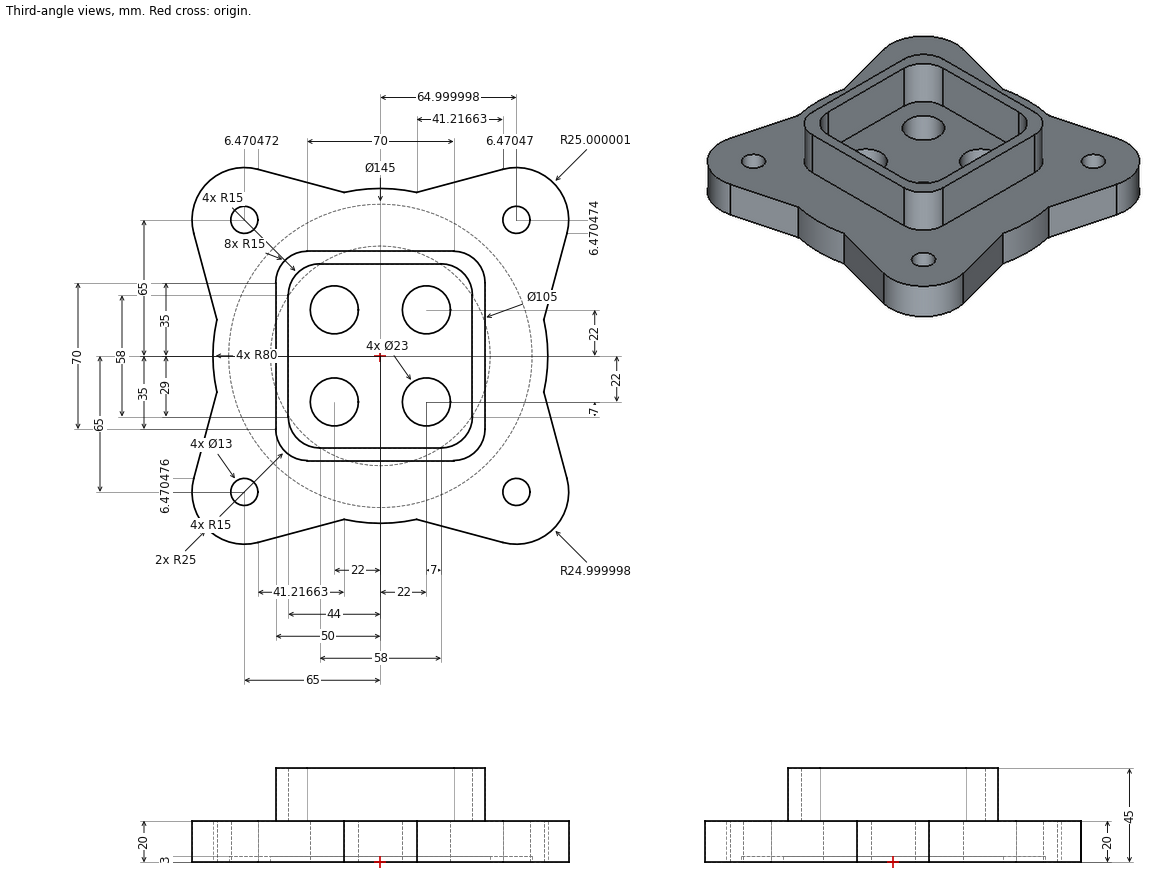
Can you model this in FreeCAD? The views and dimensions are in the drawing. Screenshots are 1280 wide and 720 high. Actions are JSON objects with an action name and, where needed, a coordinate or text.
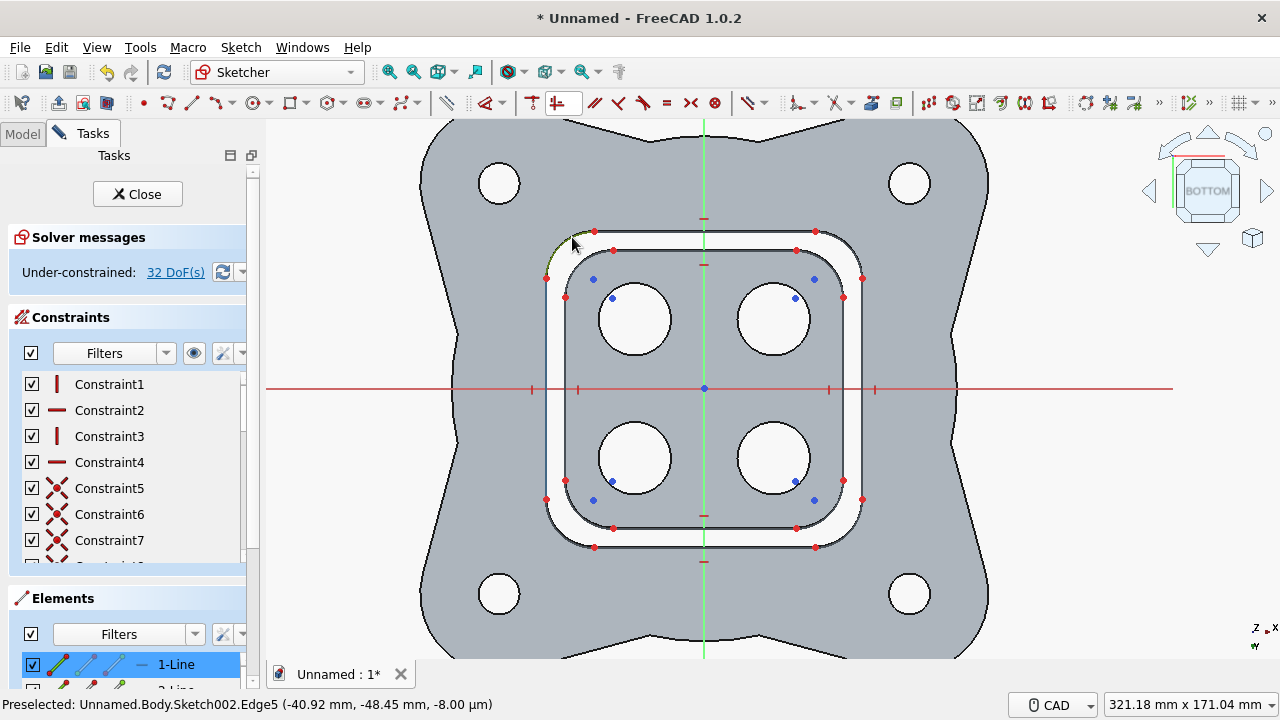
{"action": "key", "text": "t"}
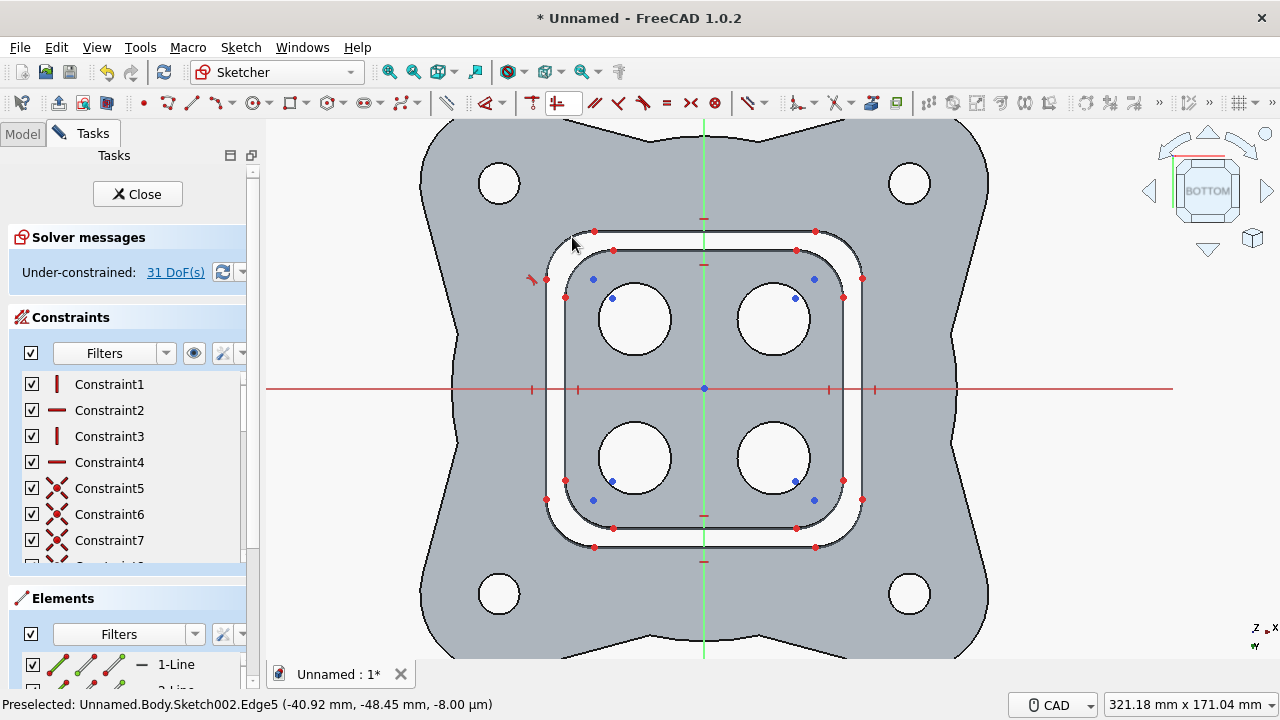
{"action": "left_click", "coordinate": [546, 434]}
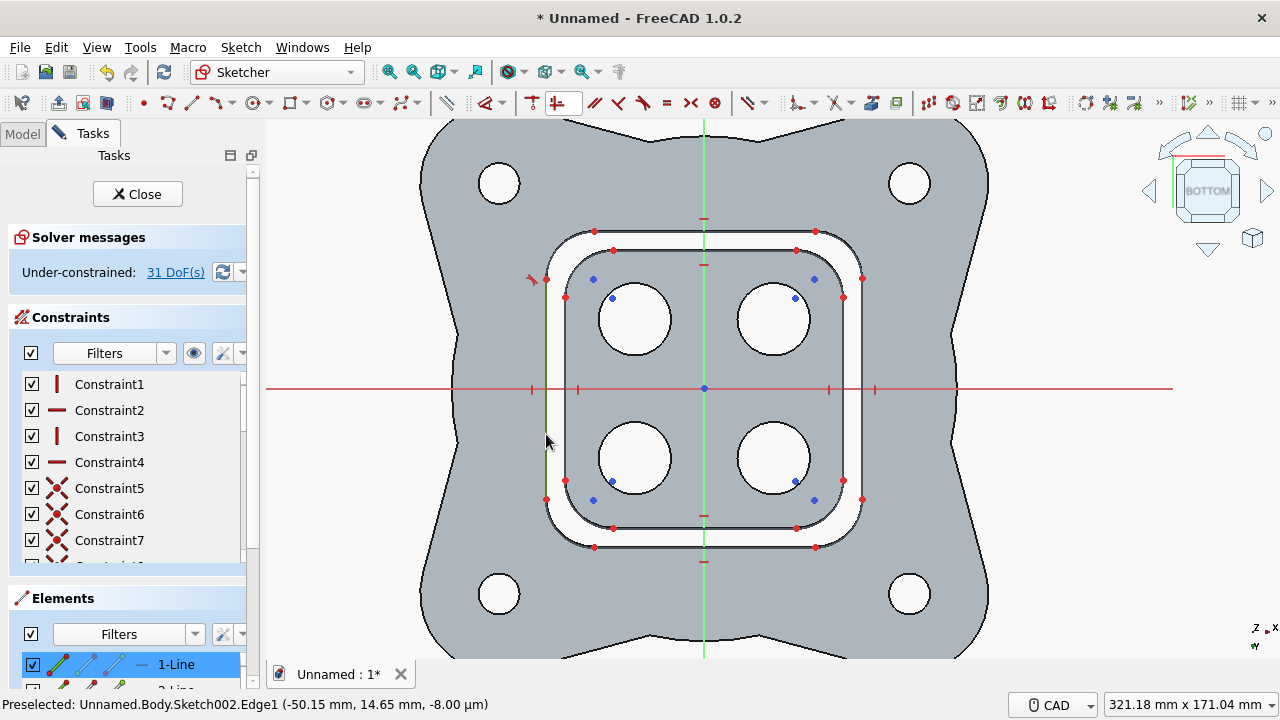
{"action": "left_click", "coordinate": [551, 522]}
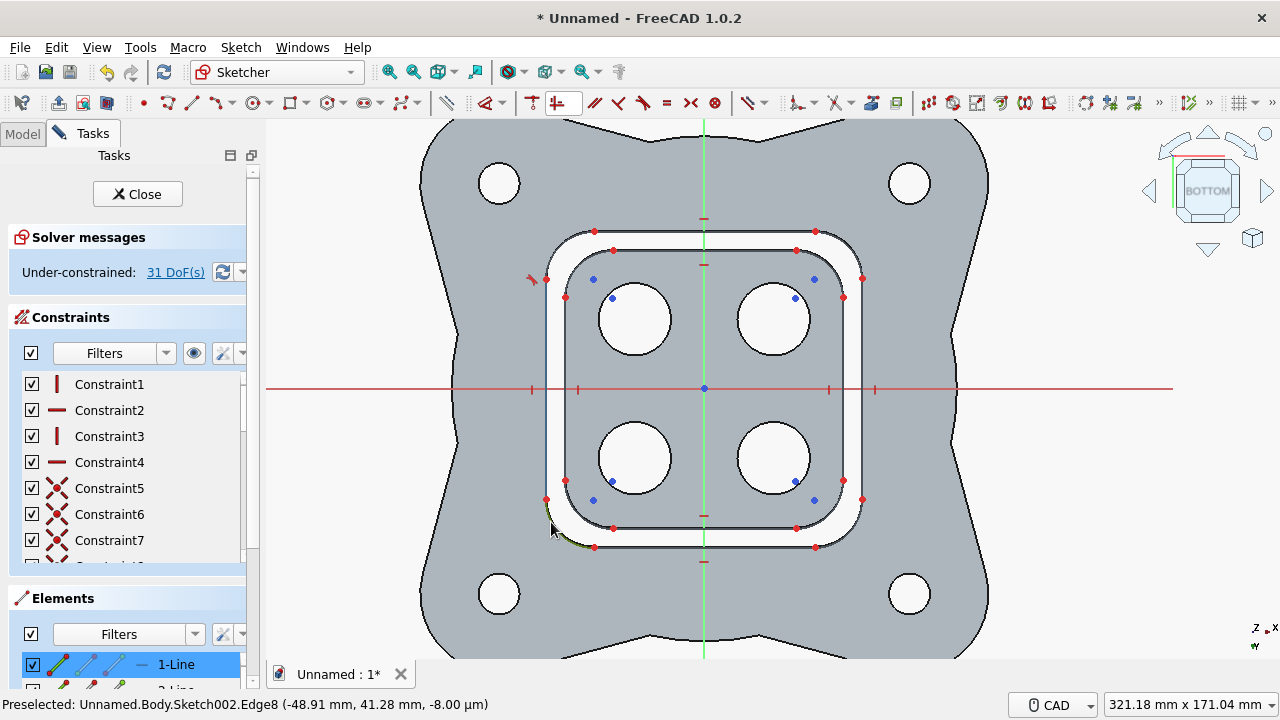
{"action": "key", "text": "t"}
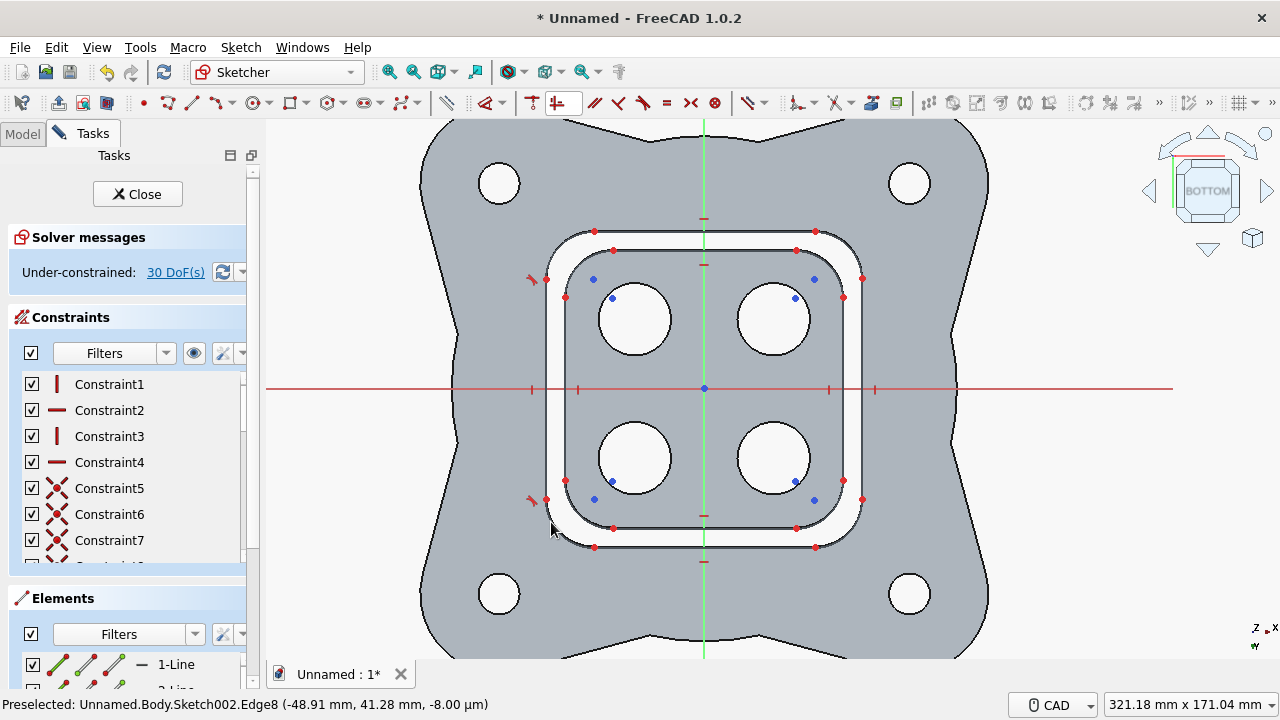
{"action": "left_click", "coordinate": [660, 232]}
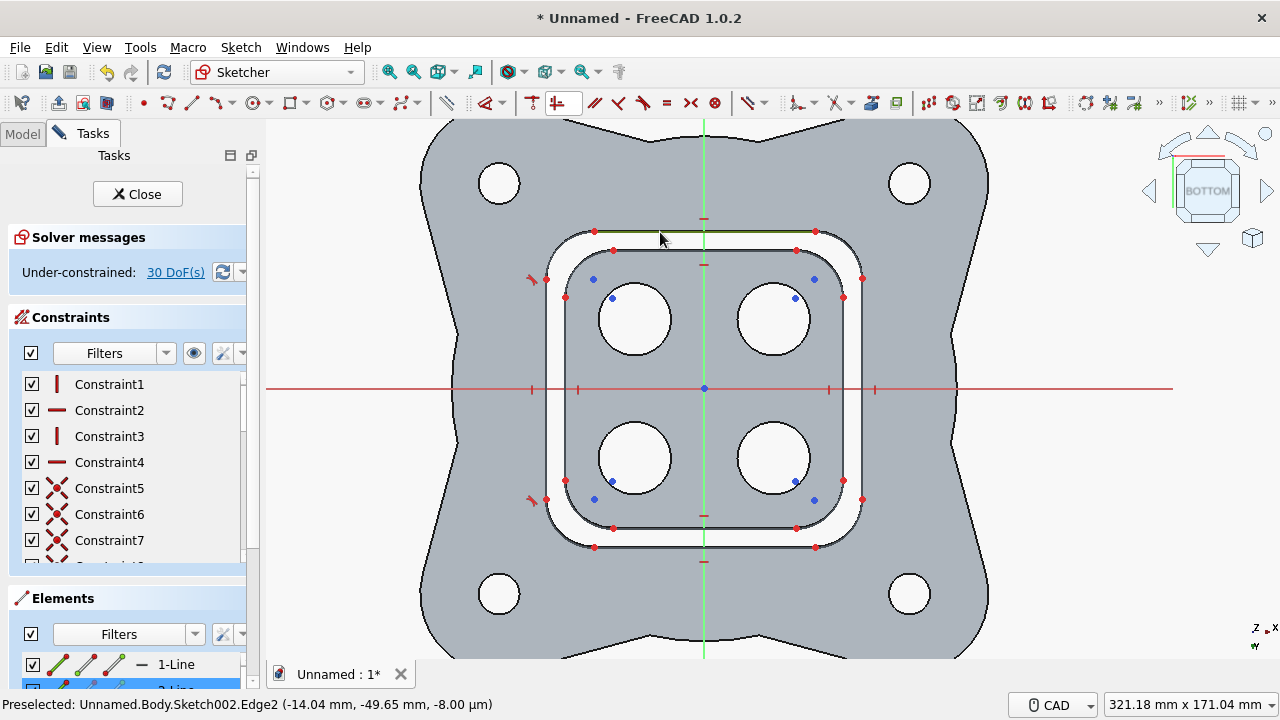
{"action": "left_click", "coordinate": [572, 237]}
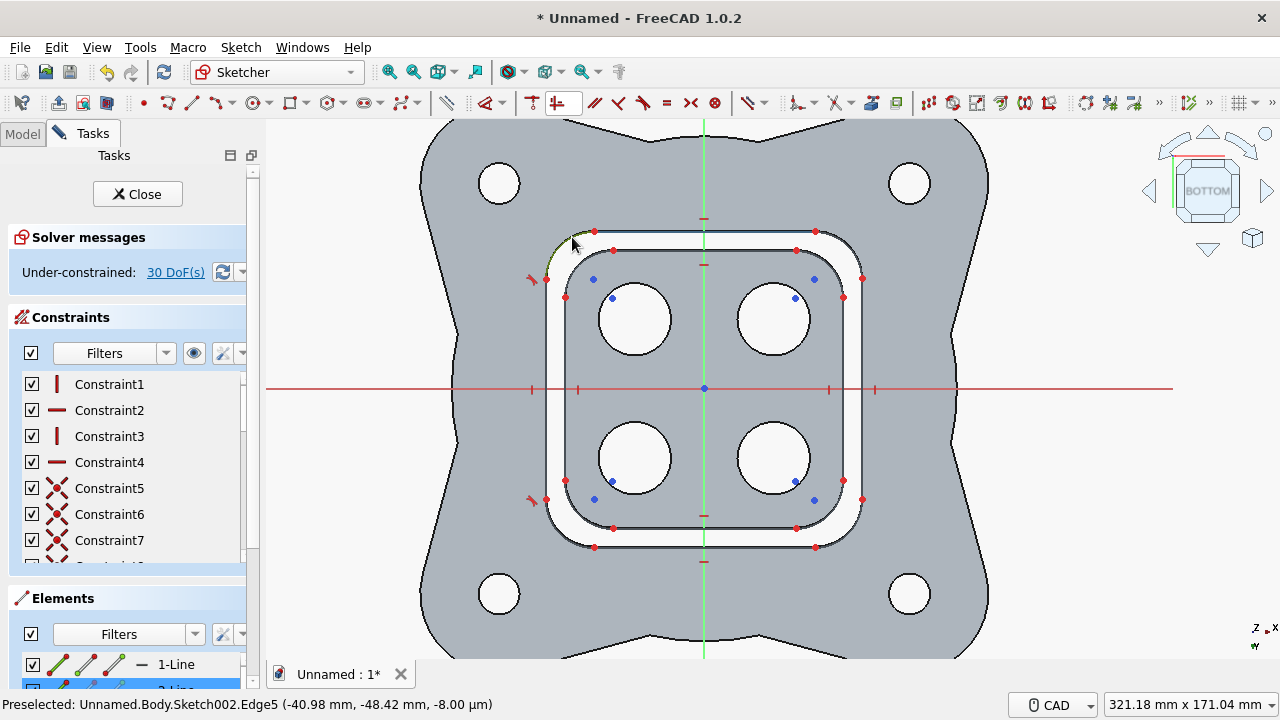
{"action": "left_click", "coordinate": [644, 104]}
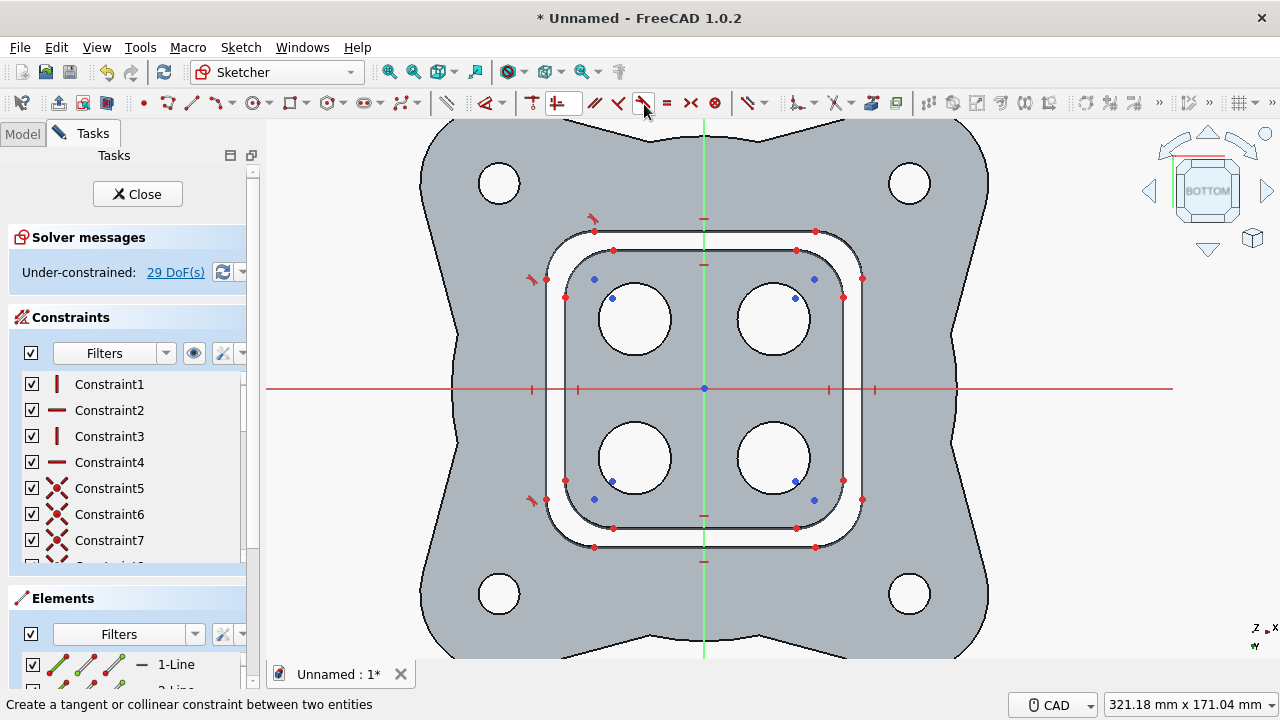
{"action": "left_click", "coordinate": [660, 232]}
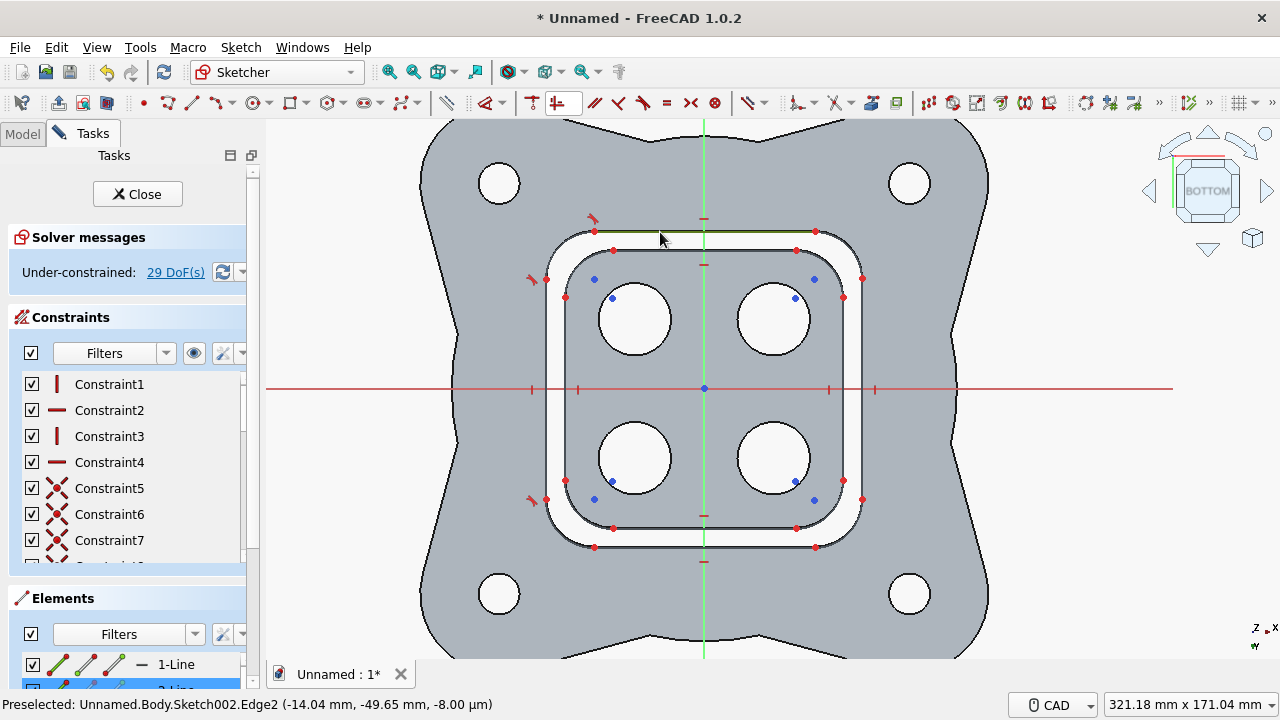
{"action": "left_click", "coordinate": [857, 258]}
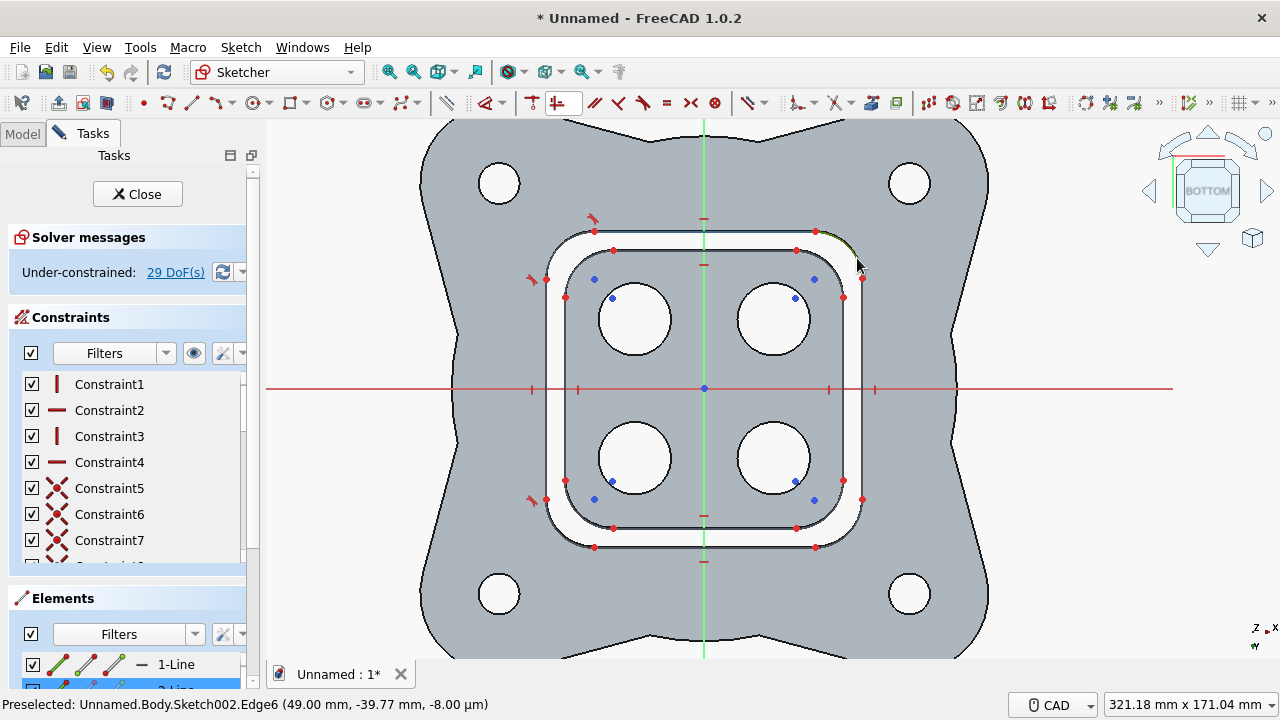
{"action": "left_click", "coordinate": [644, 104]}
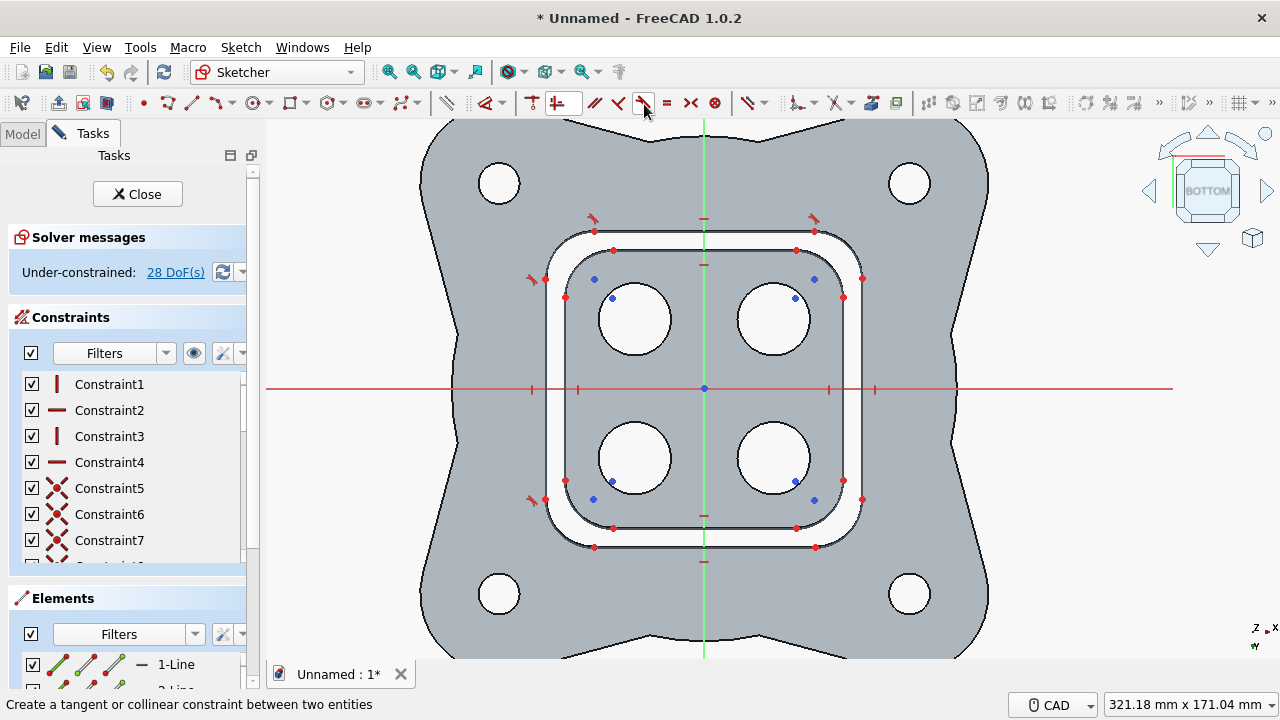
{"action": "left_click", "coordinate": [862, 345]}